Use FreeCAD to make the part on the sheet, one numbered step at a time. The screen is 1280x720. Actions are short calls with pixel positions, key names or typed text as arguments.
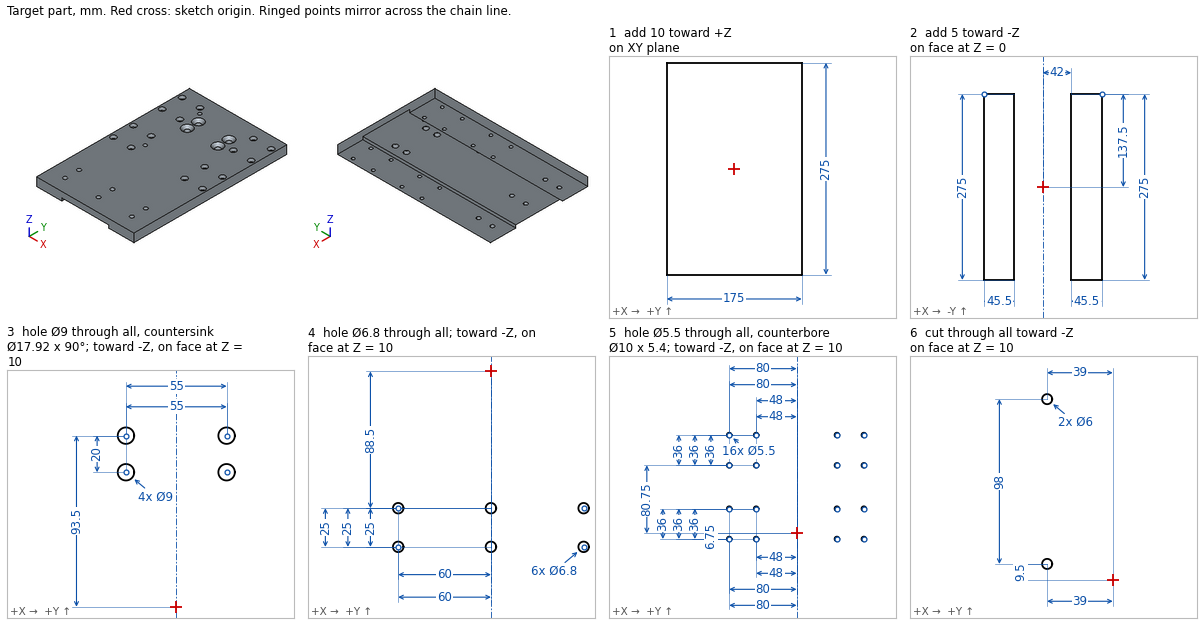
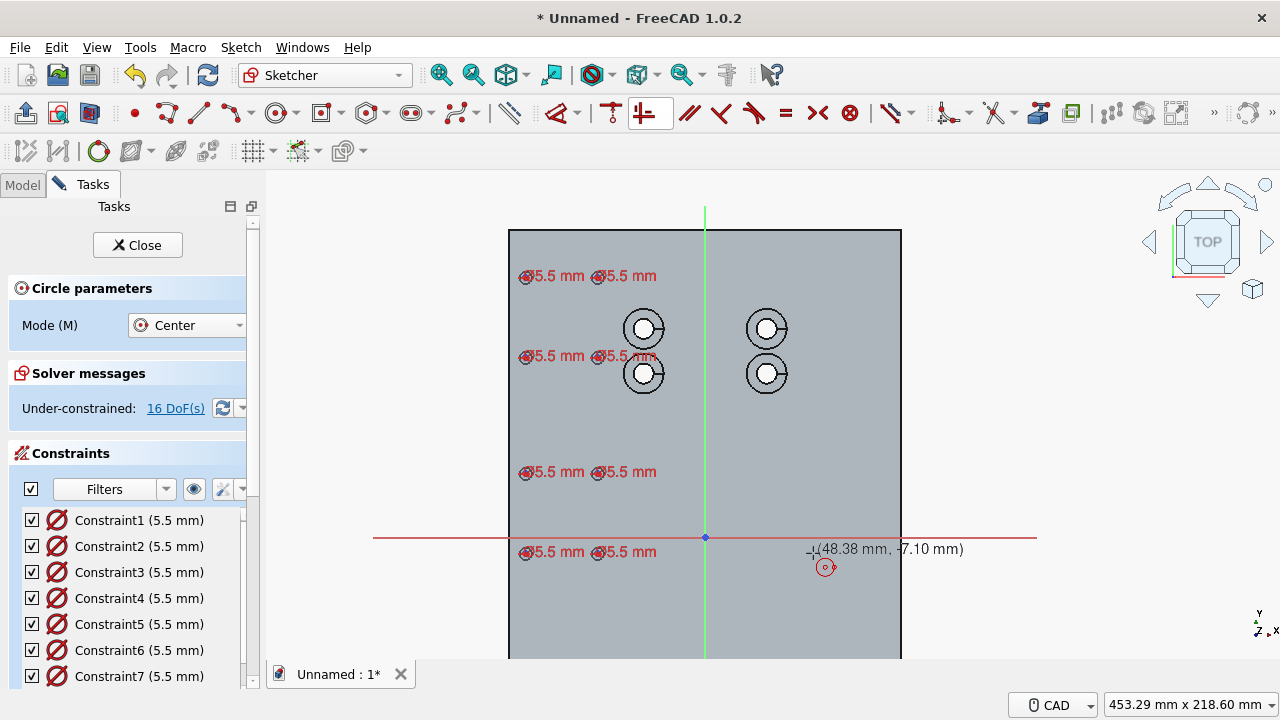
click(813, 553)
move(817, 557)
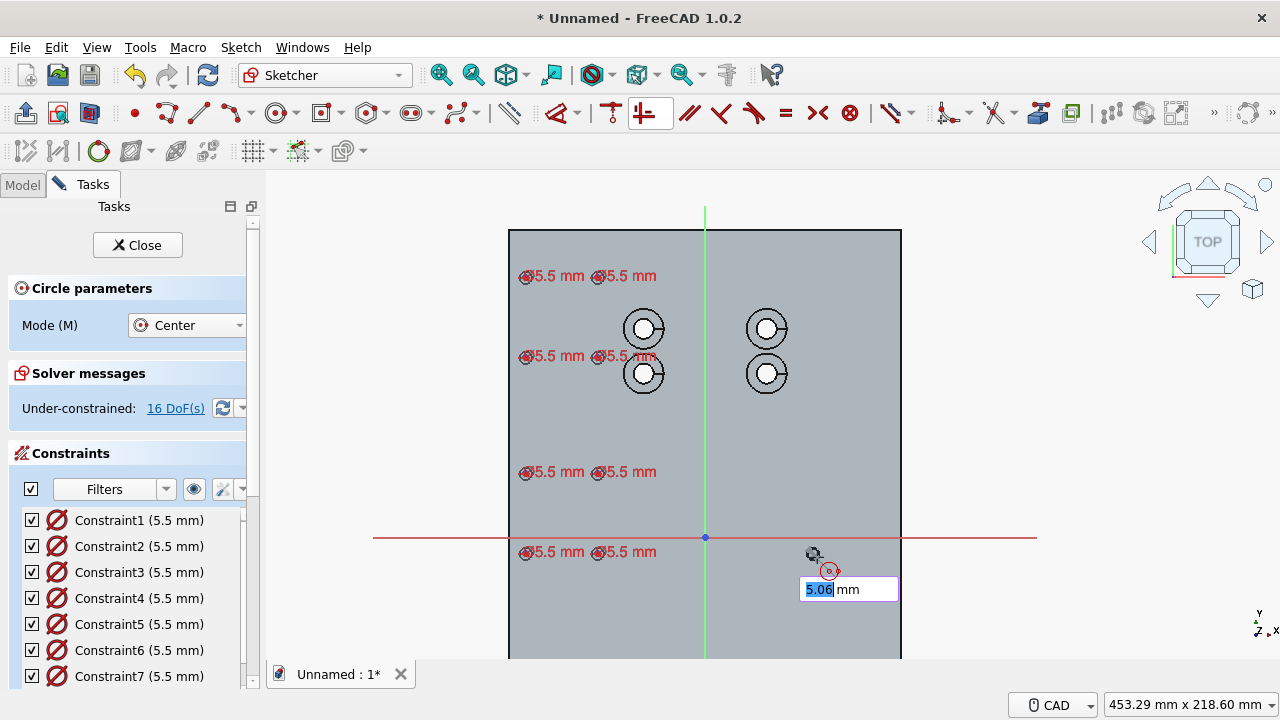
text(5.5)
key(Return)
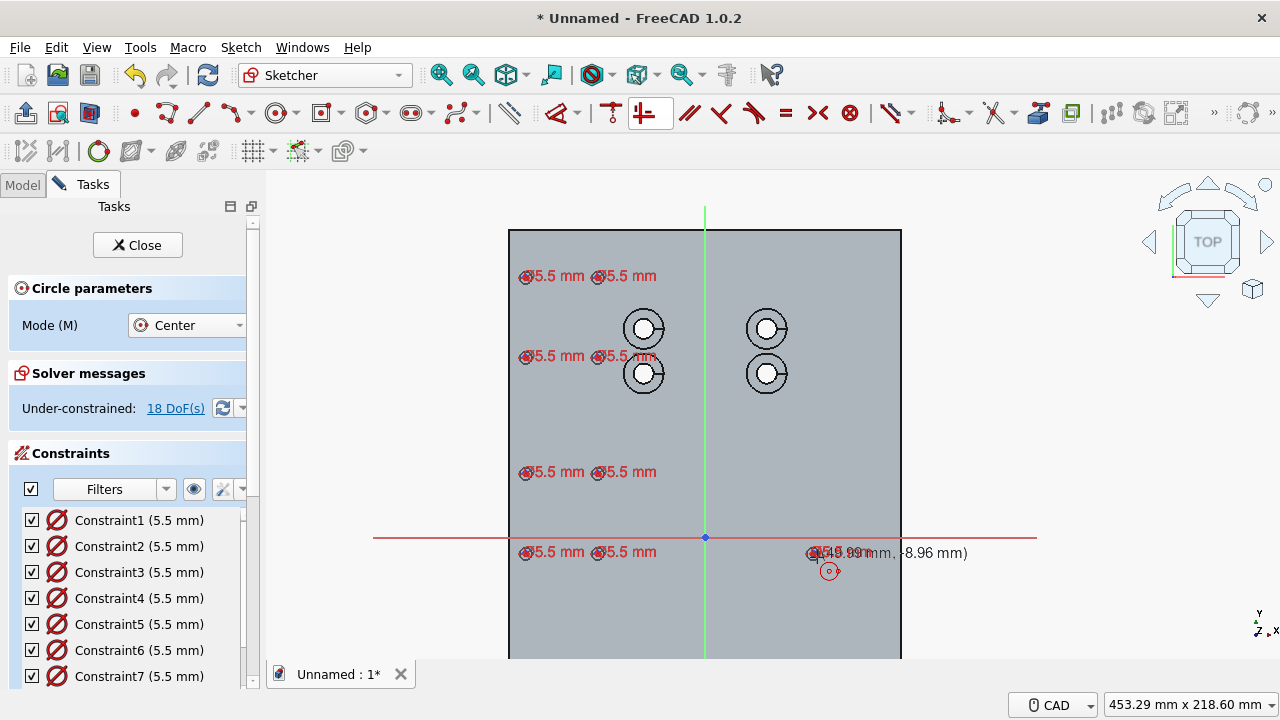
scroll(884, 553, up, 7)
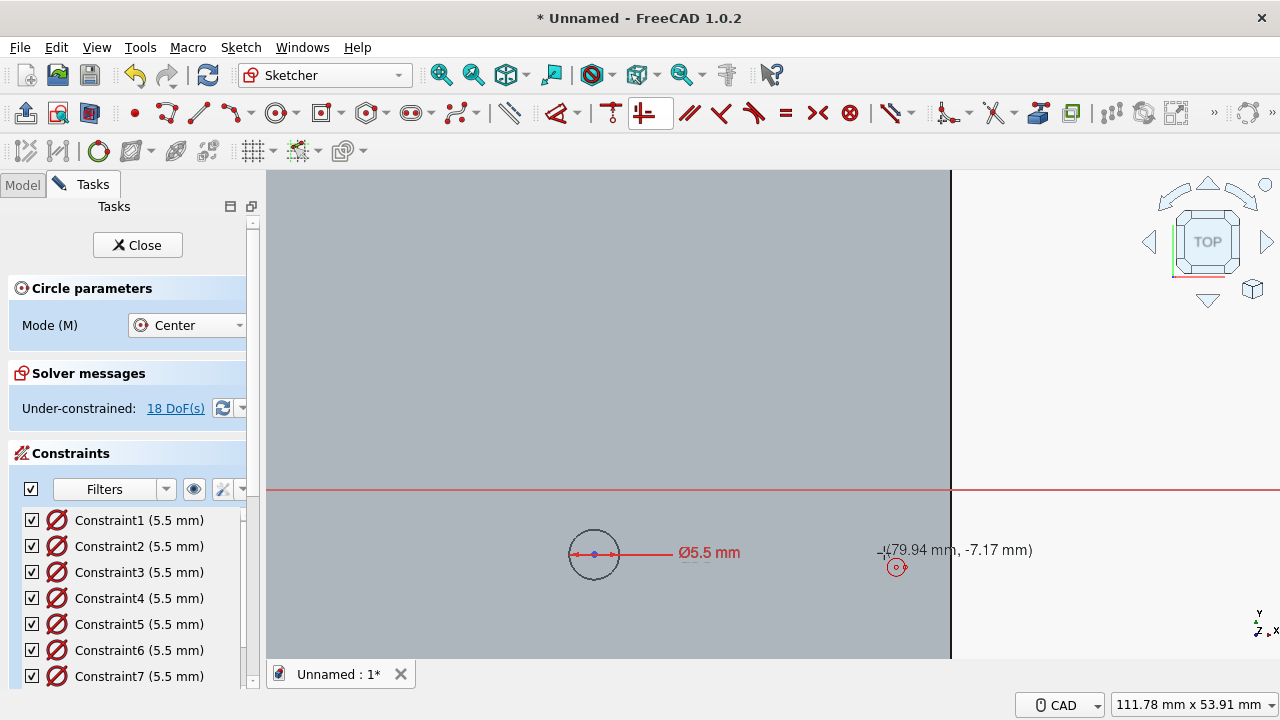
scroll(884, 553, down, 7)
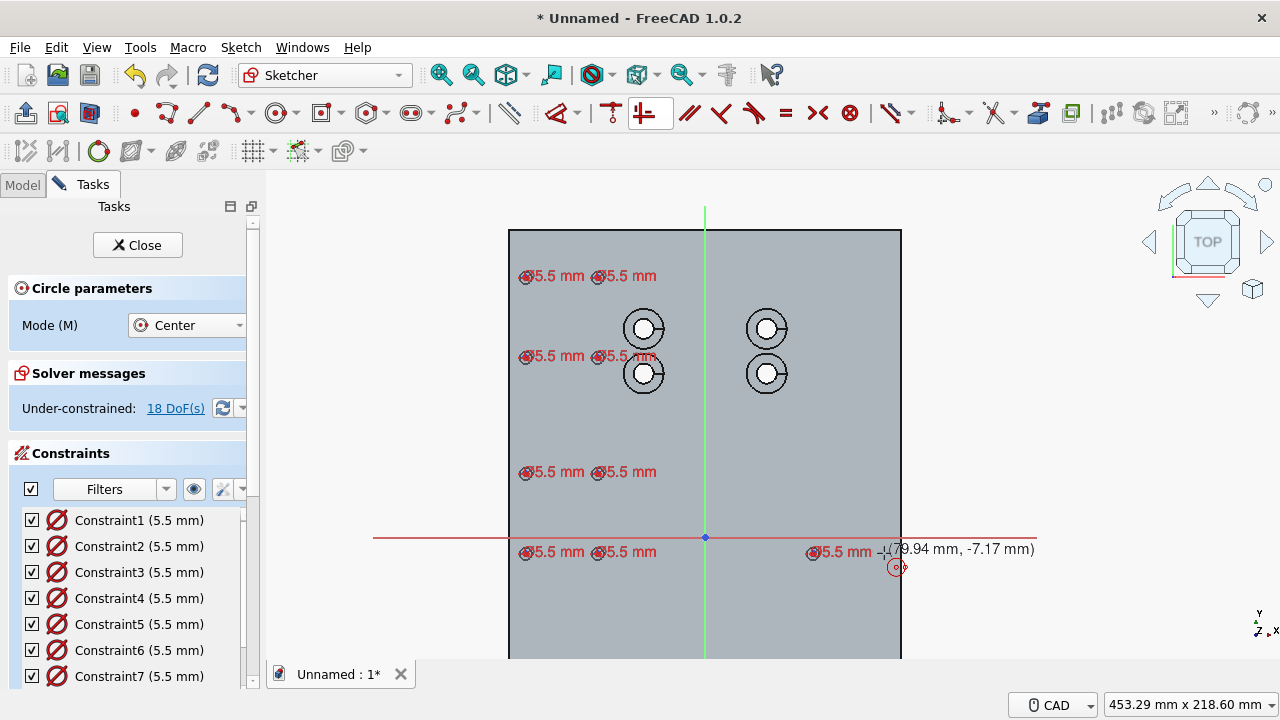
click(884, 553)
move(888, 557)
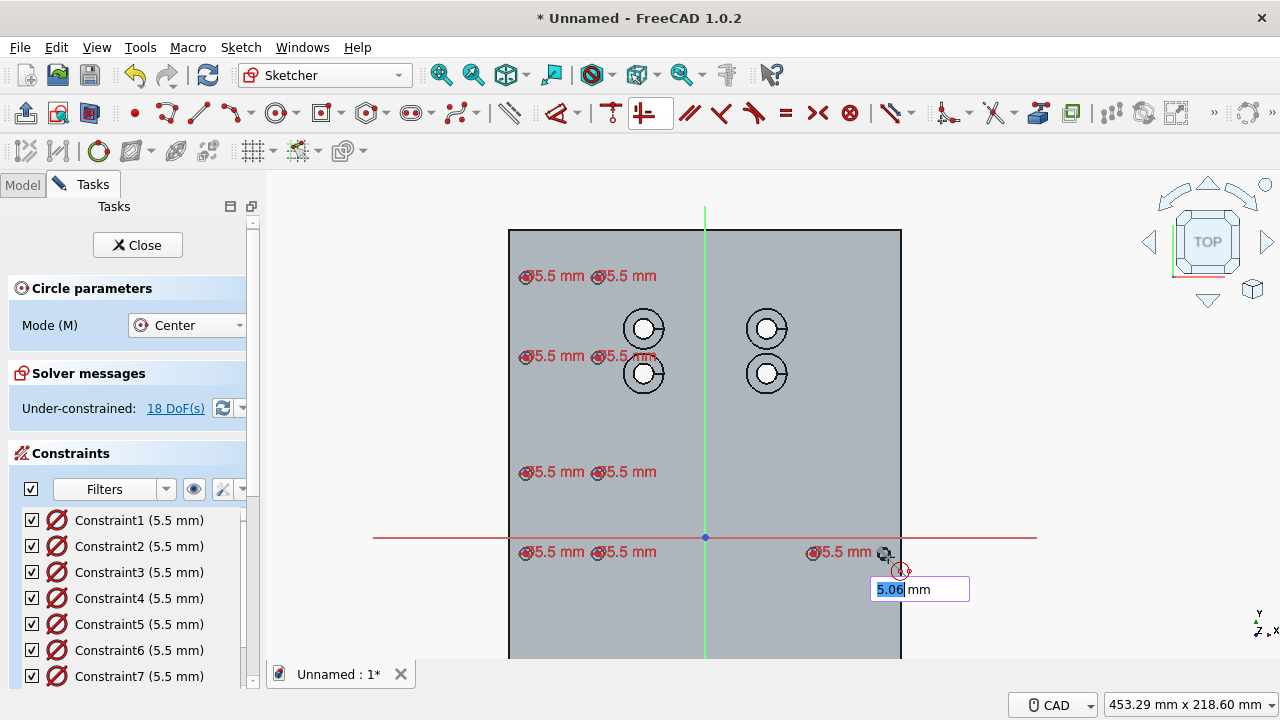
text(5.5)
key(Return)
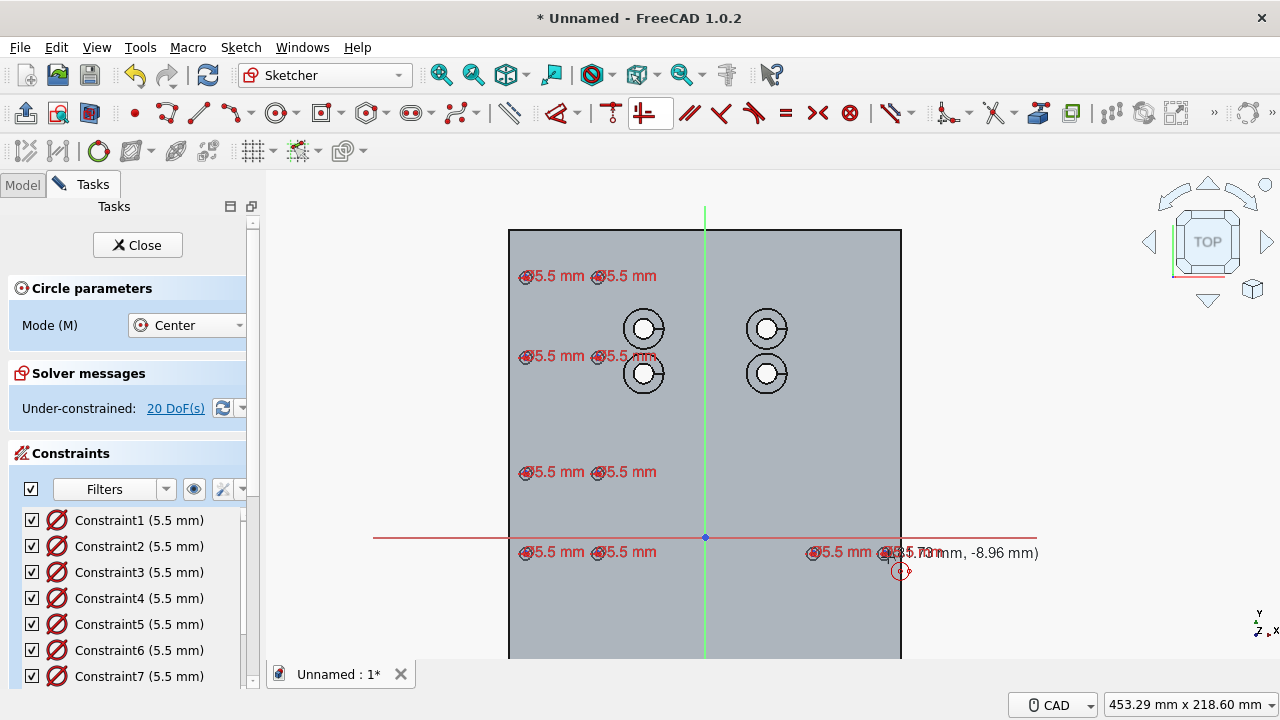
scroll(813, 473, up, 7)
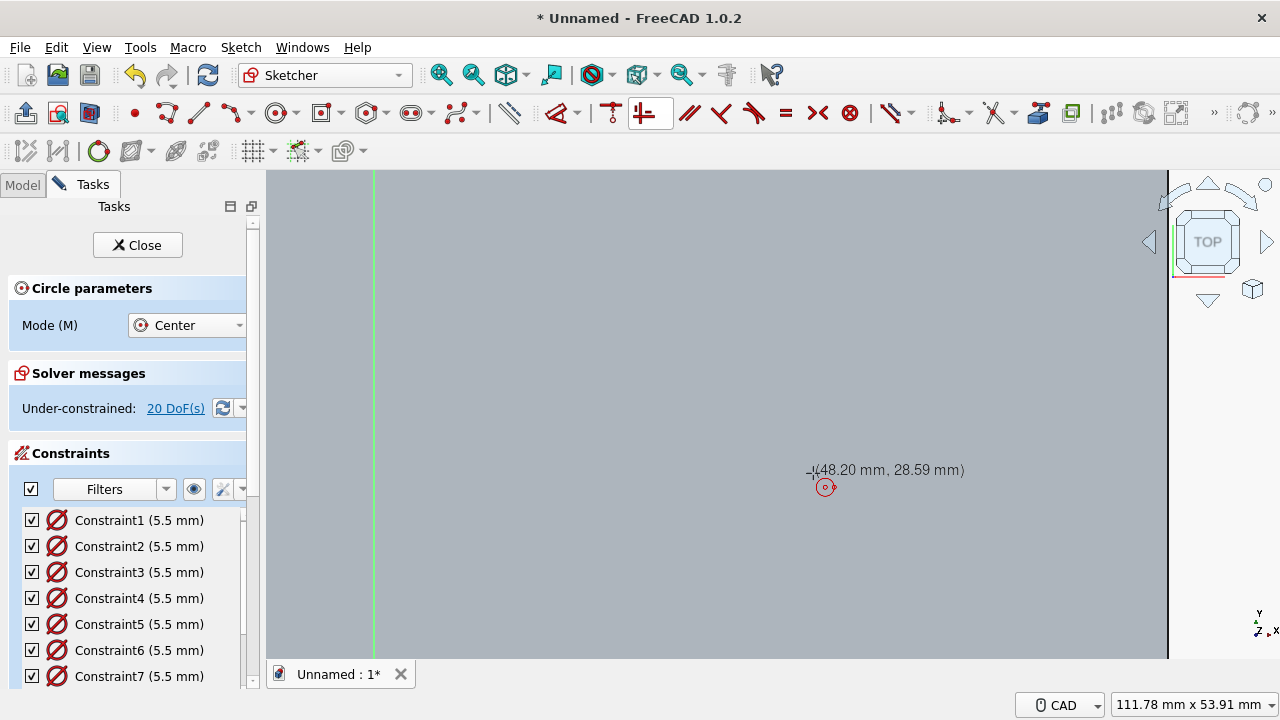
scroll(813, 473, down, 7)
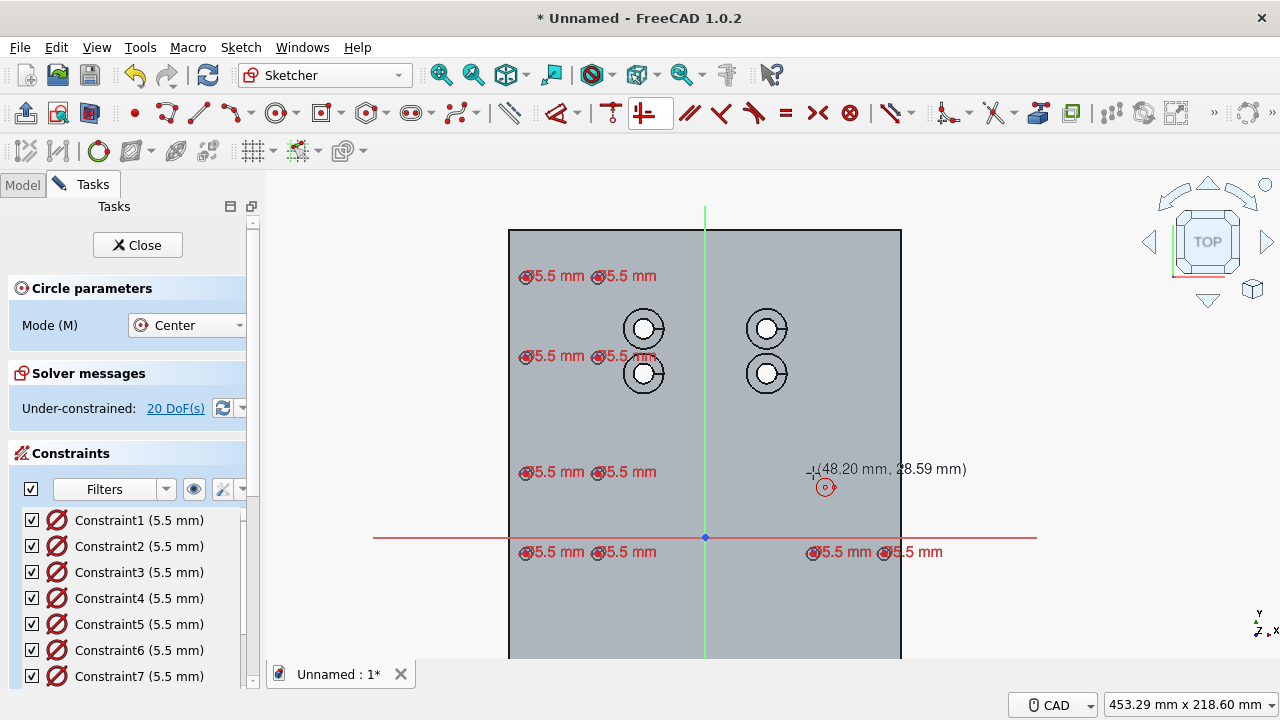
click(813, 473)
move(817, 468)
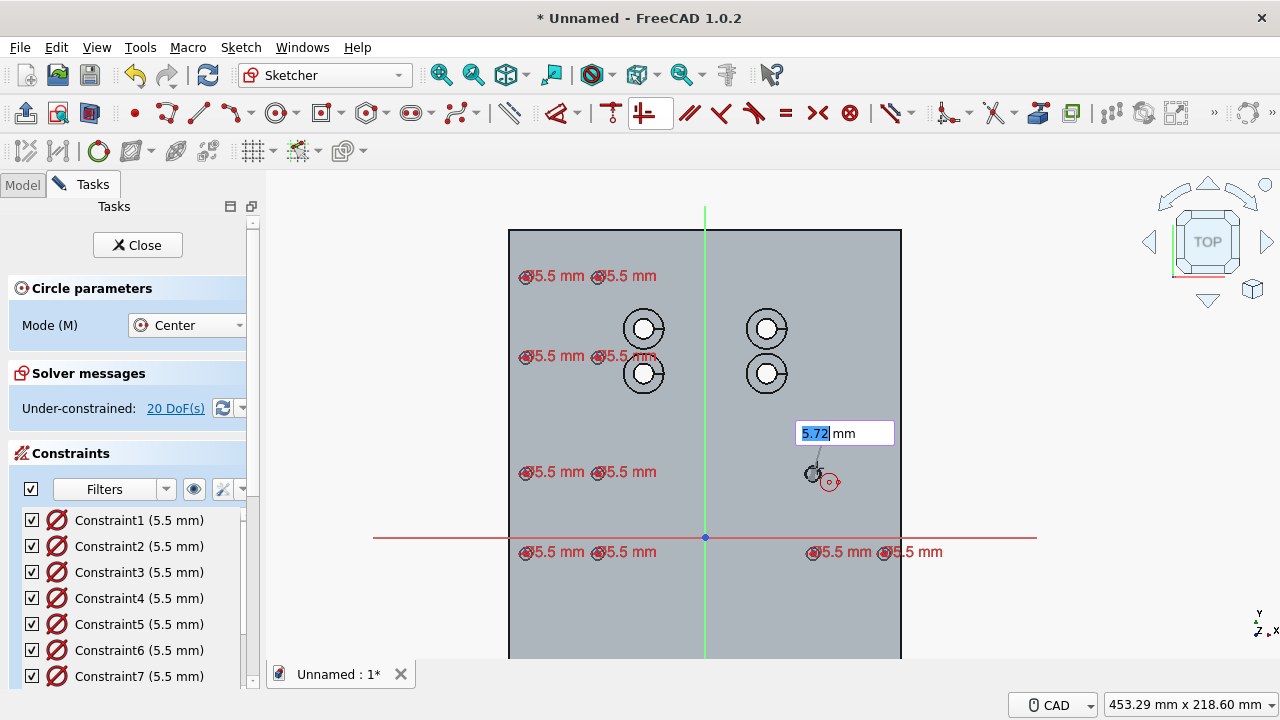
text(5.5)
key(Return)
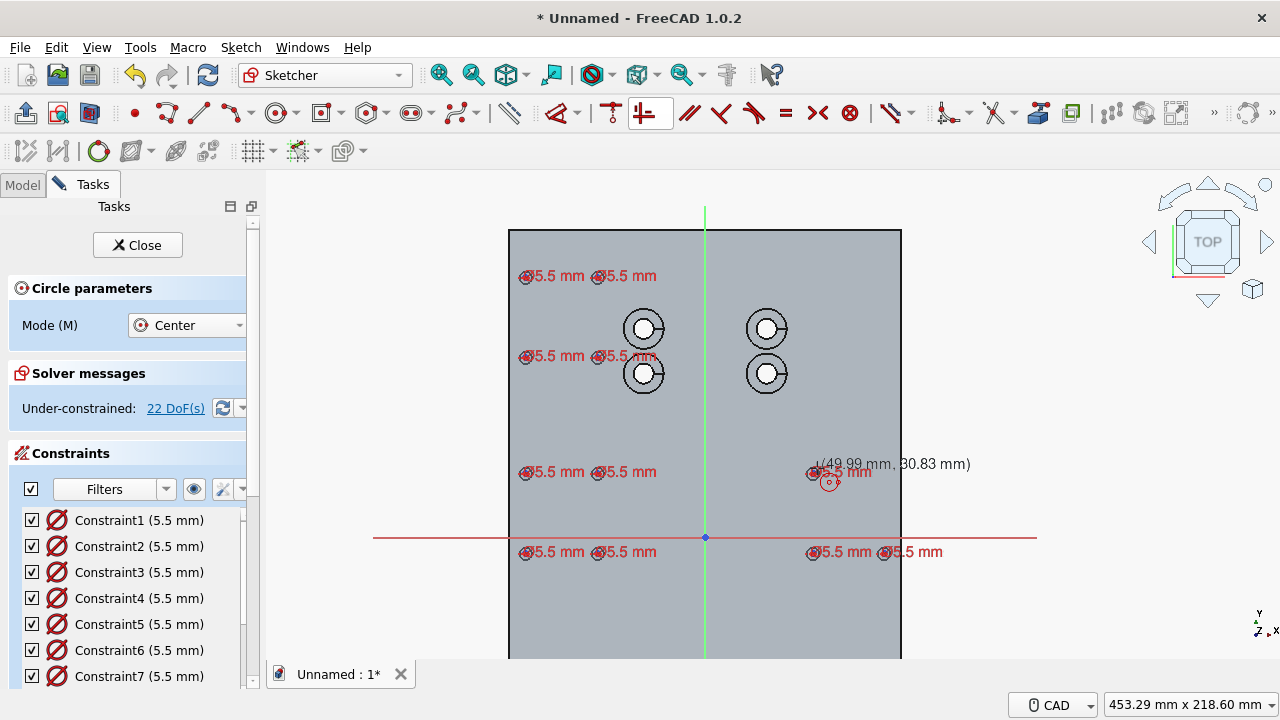
scroll(884, 473, up, 7)